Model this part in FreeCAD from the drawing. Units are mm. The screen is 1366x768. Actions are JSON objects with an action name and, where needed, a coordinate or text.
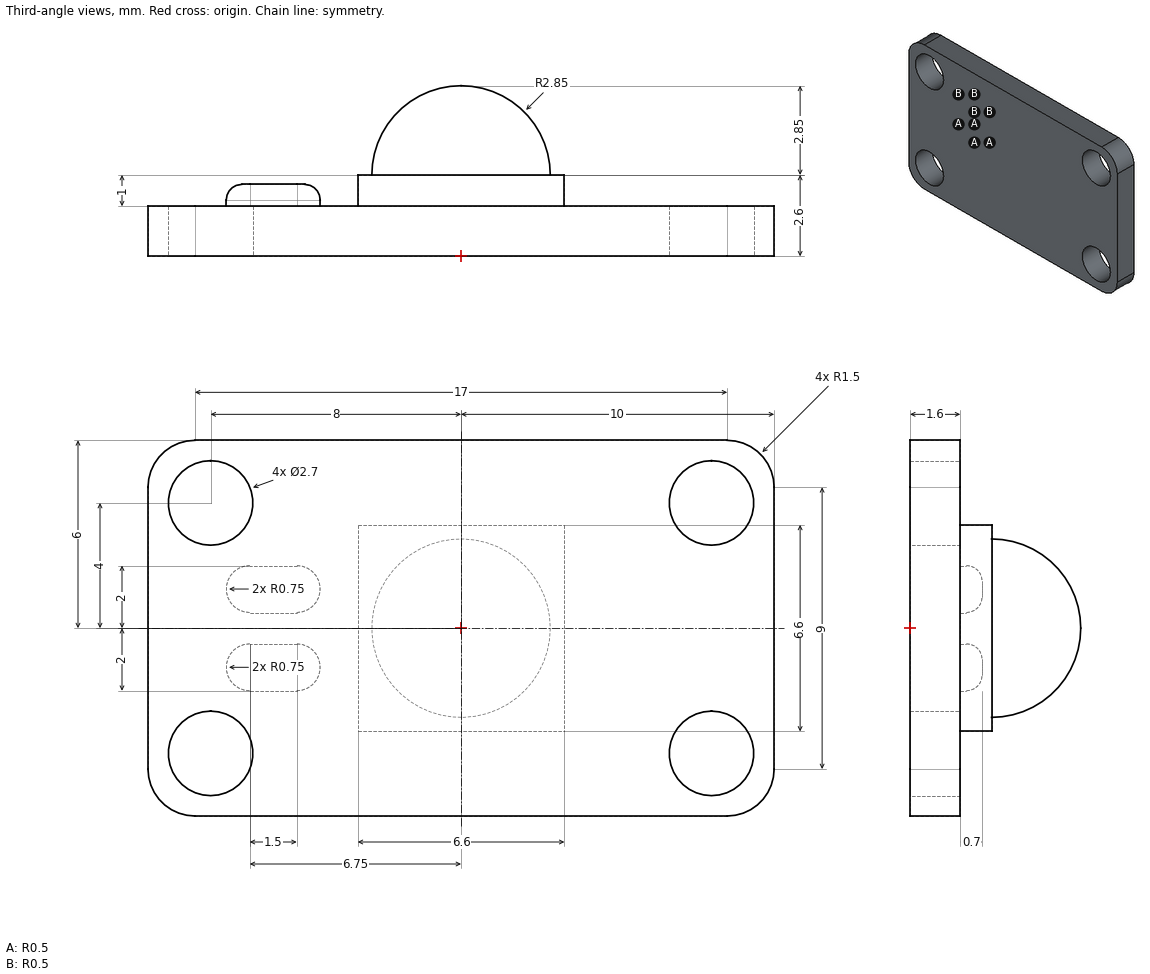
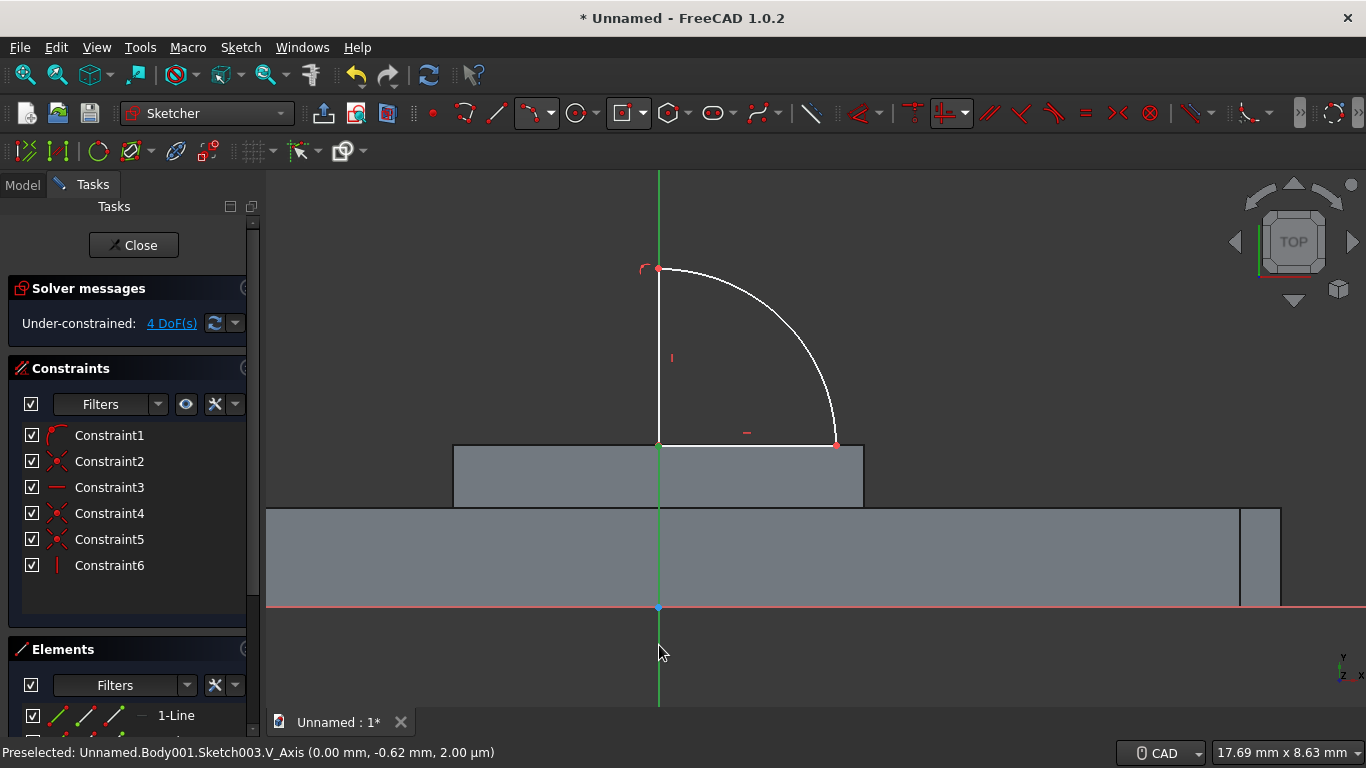
{"action": "left_click", "coordinate": [914, 114]}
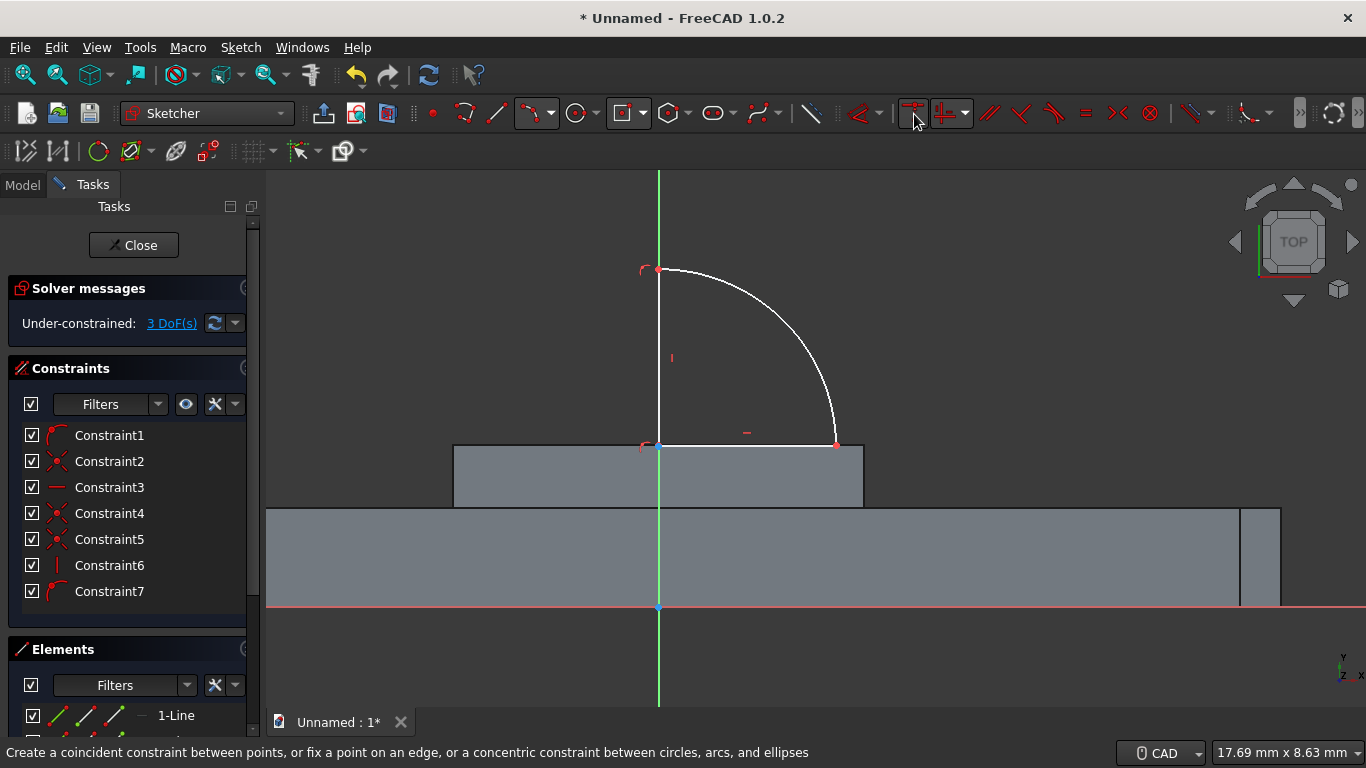
{"action": "left_click", "coordinate": [858, 114]}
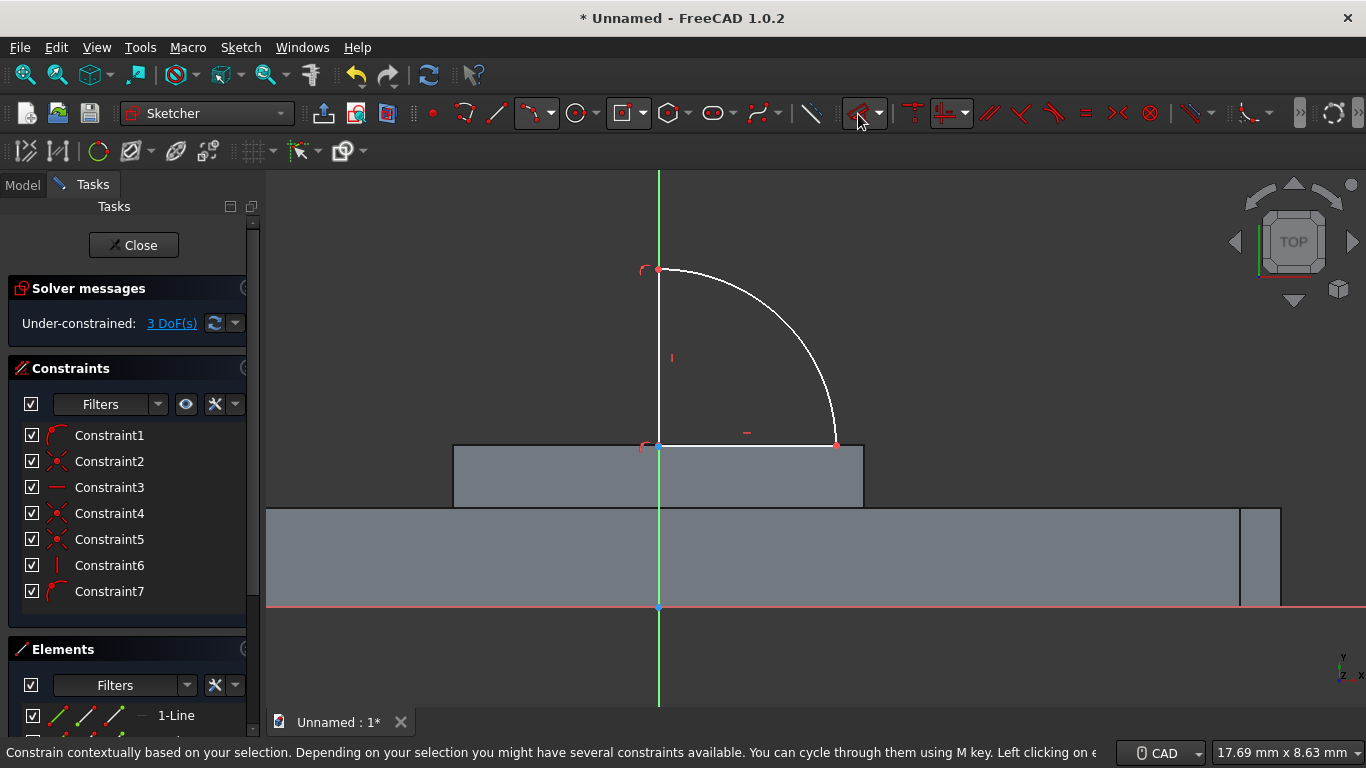
{"action": "left_click", "coordinate": [816, 366]}
{"action": "left_click", "coordinate": [844, 351]}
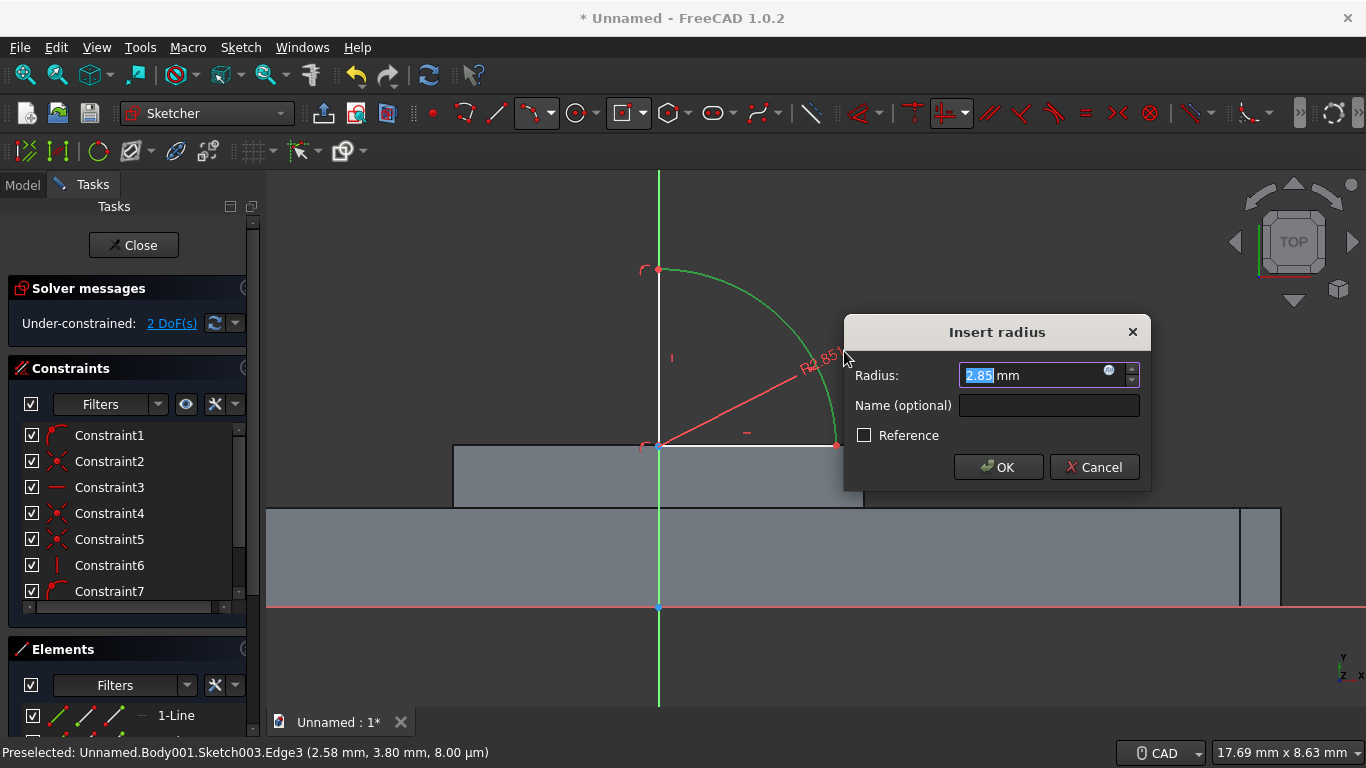
{"action": "type", "text": "2.85"}
{"action": "key", "text": "Return"}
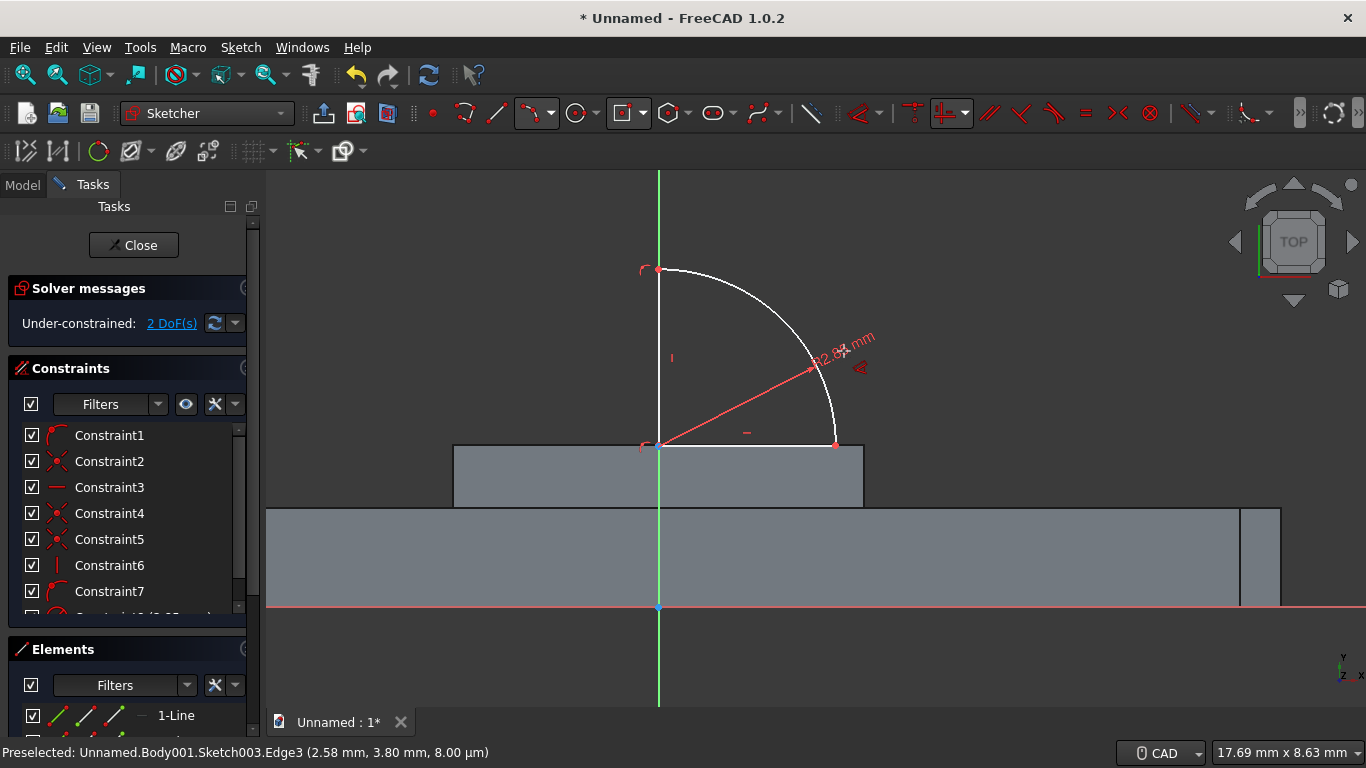
{"action": "left_click", "coordinate": [659, 322]}
{"action": "left_click", "coordinate": [625, 358]}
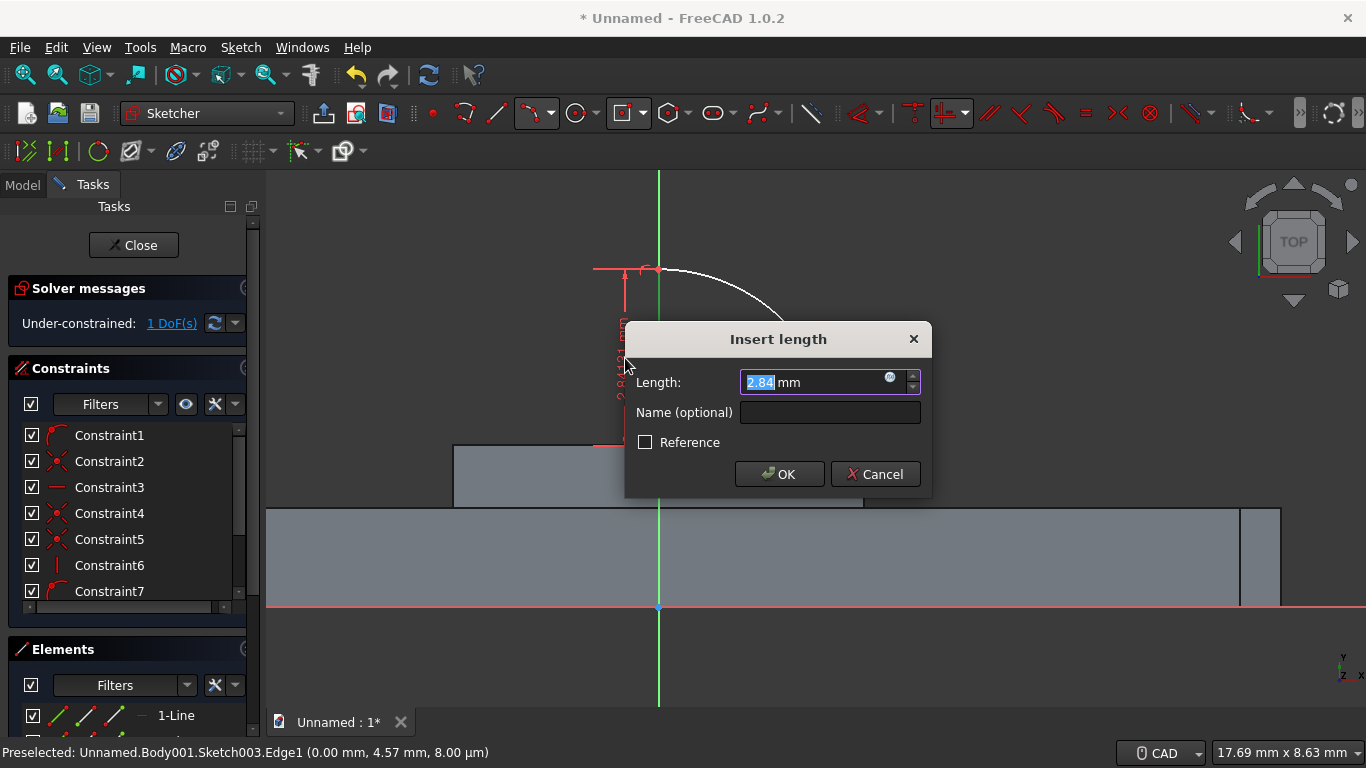
{"action": "type", "text": "2.85"}
{"action": "key", "text": "Return"}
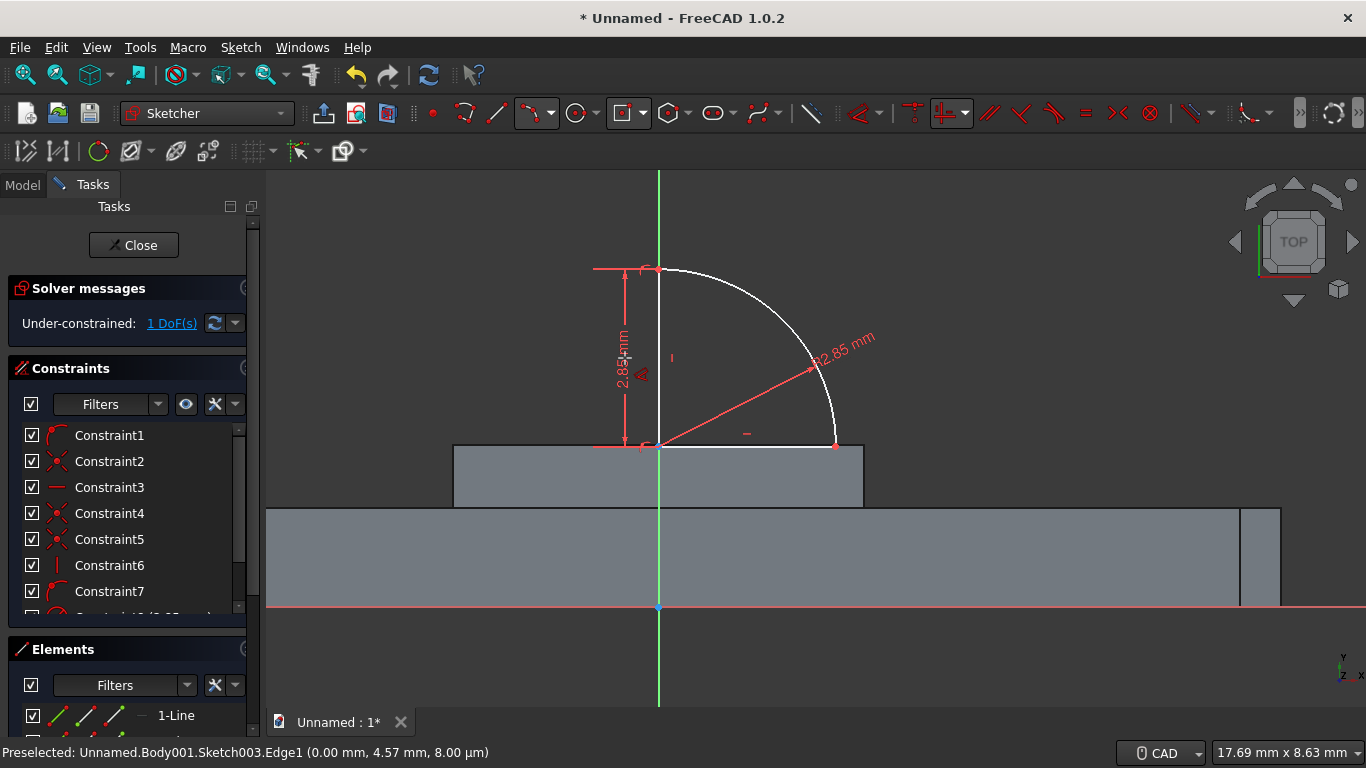
{"action": "left_click", "coordinate": [659, 447]}
{"action": "left_click", "coordinate": [625, 527]}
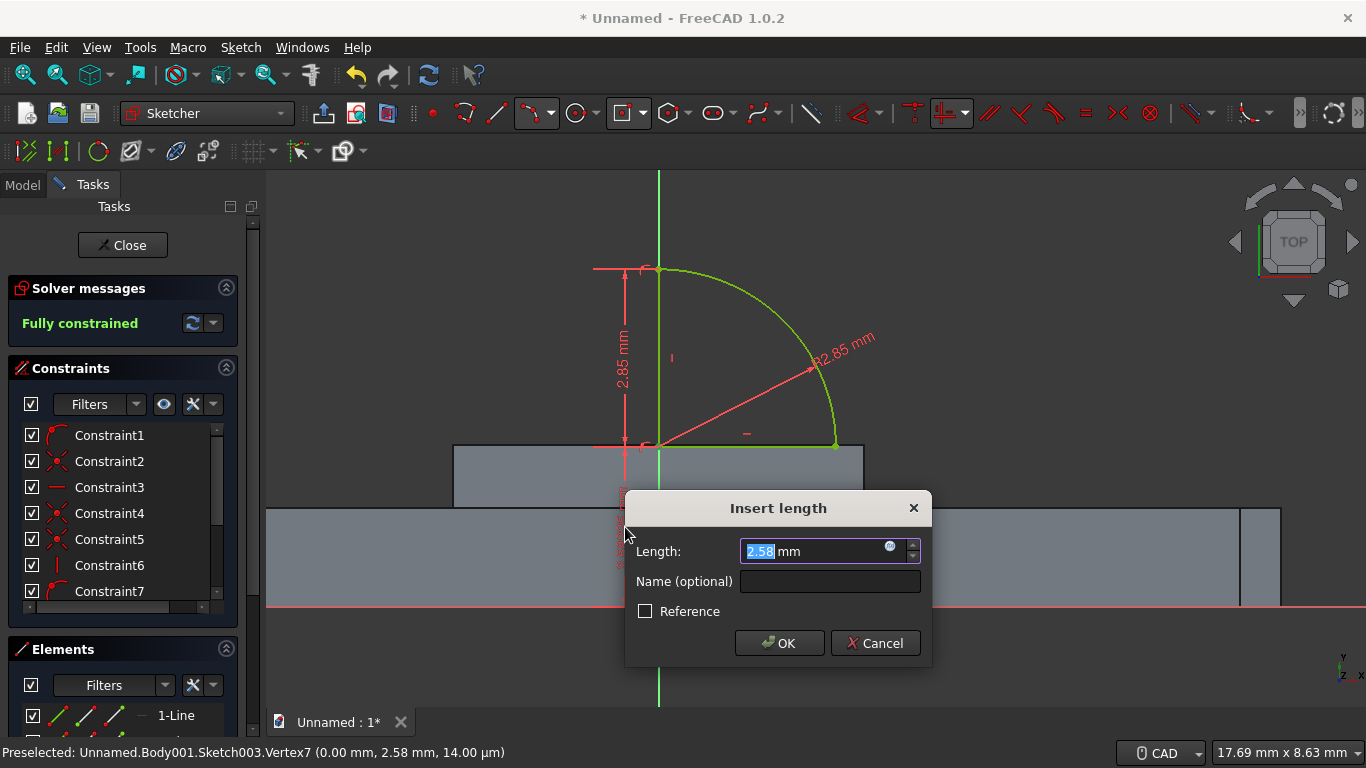
{"action": "type", "text": "2.6"}
{"action": "key", "text": "Return"}
{"action": "key", "text": "Escape"}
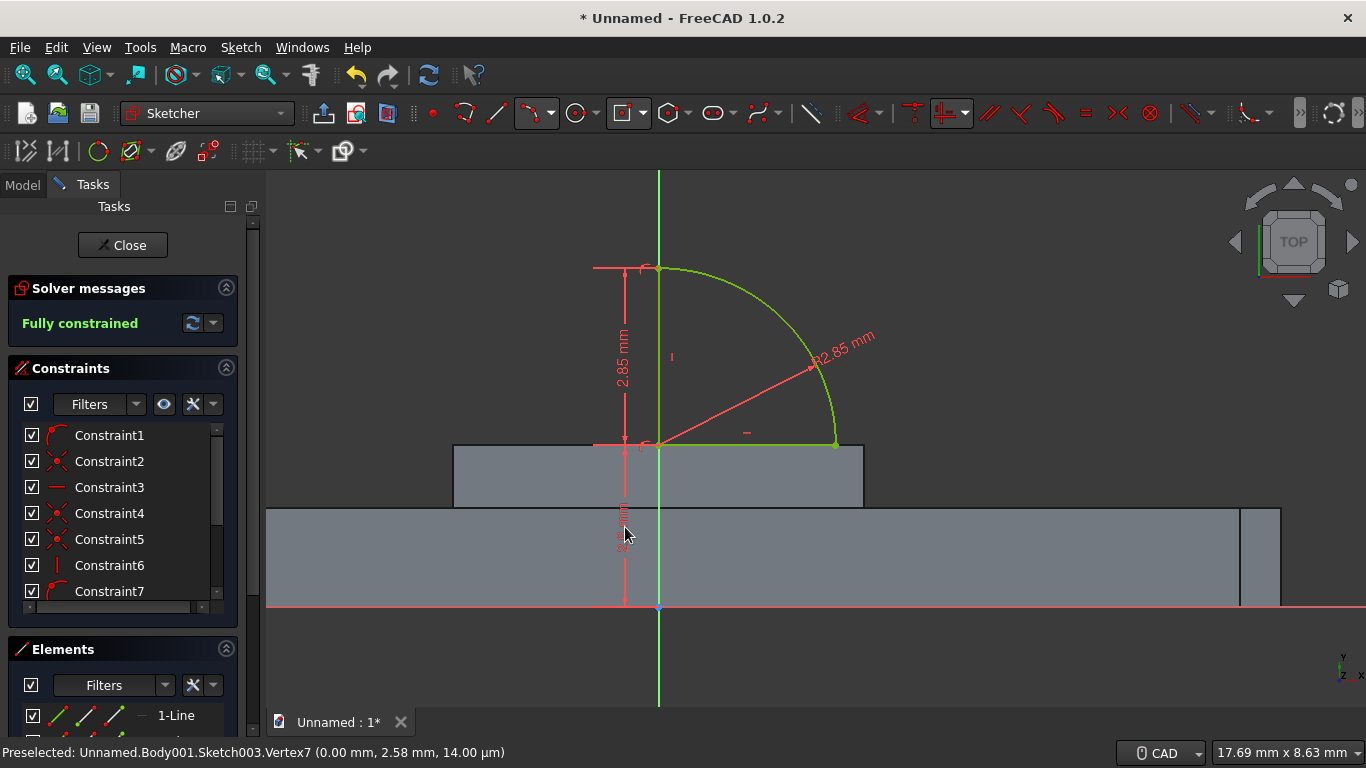
{"action": "left_click", "coordinate": [123, 245]}